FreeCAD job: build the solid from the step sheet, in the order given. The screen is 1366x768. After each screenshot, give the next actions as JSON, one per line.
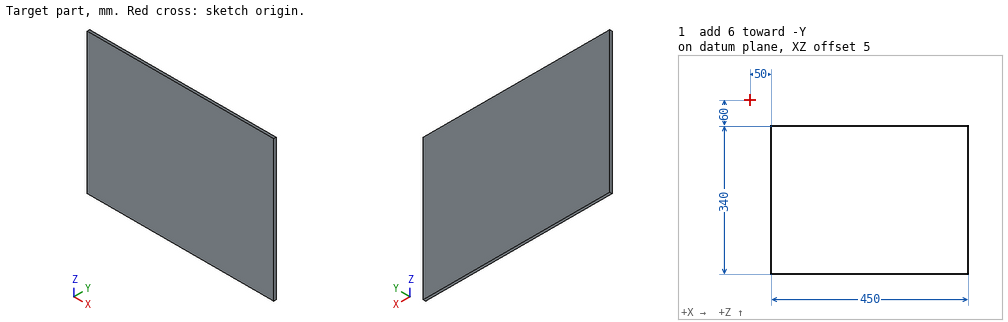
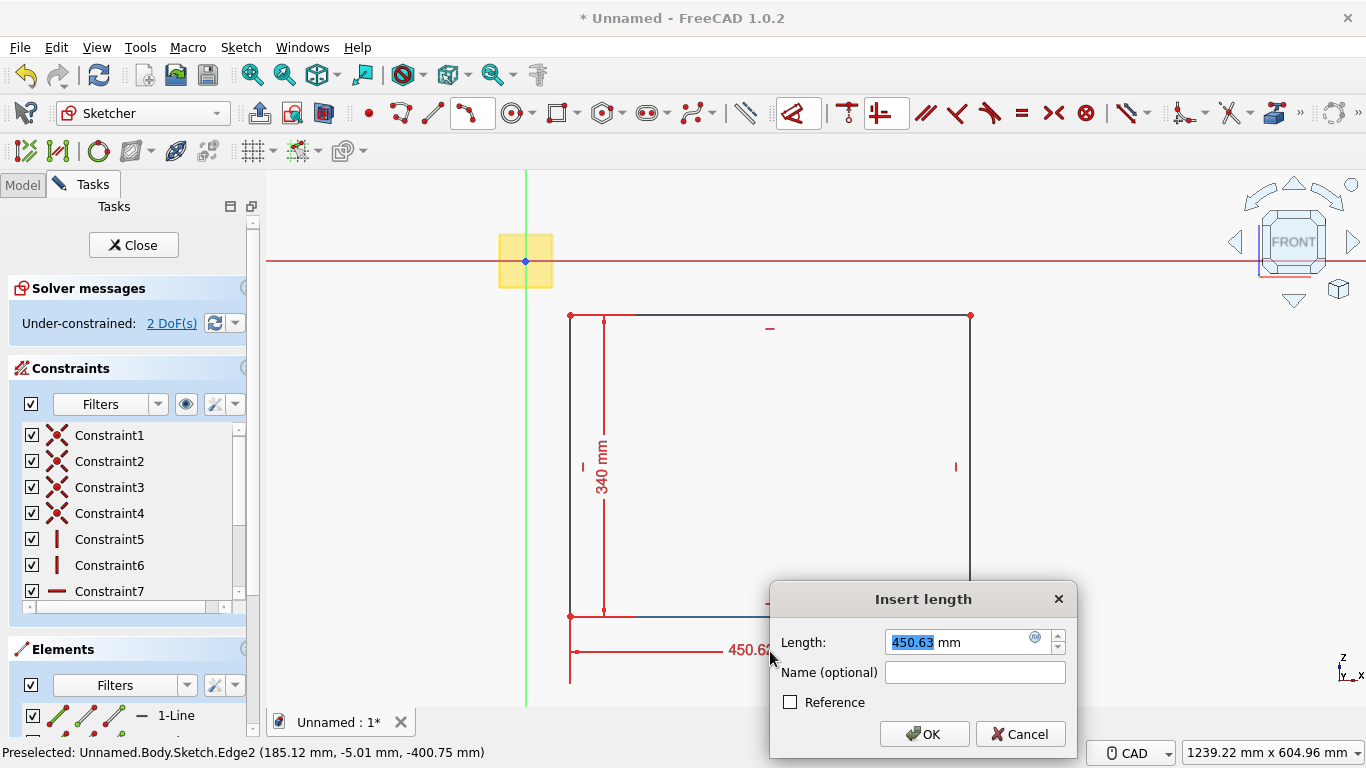
{"action": "type", "text": "450"}
{"action": "key", "text": "Return"}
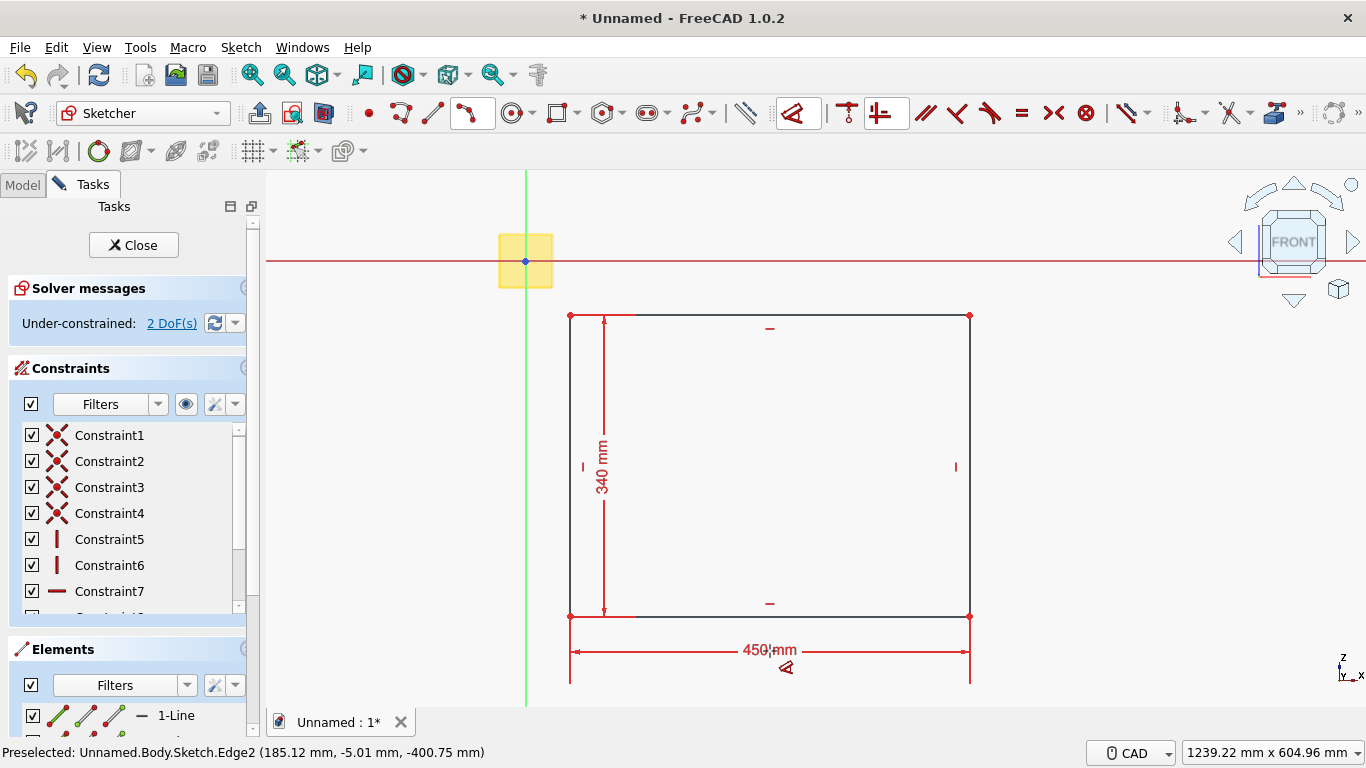
{"action": "left_click", "coordinate": [570, 315]}
{"action": "left_click", "coordinate": [548, 227]}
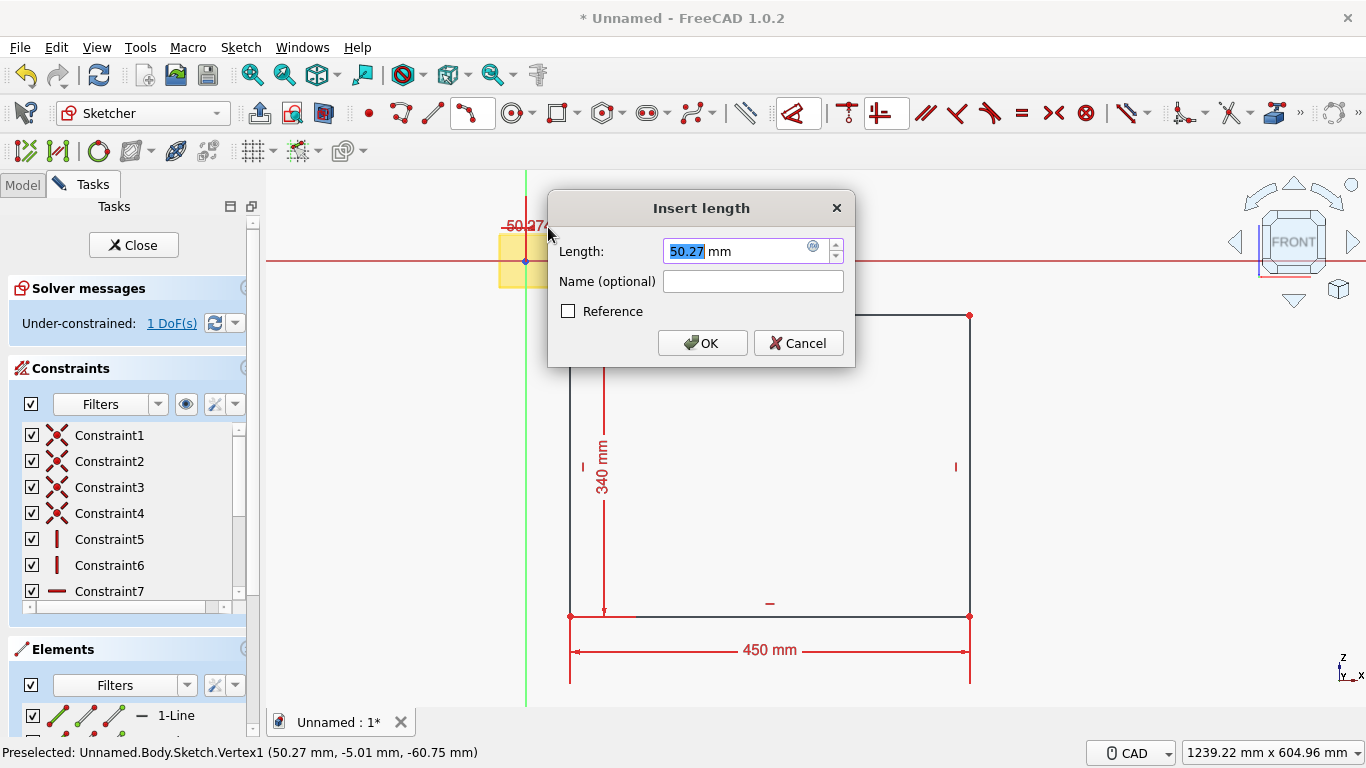
{"action": "type", "text": "50"}
{"action": "key", "text": "Return"}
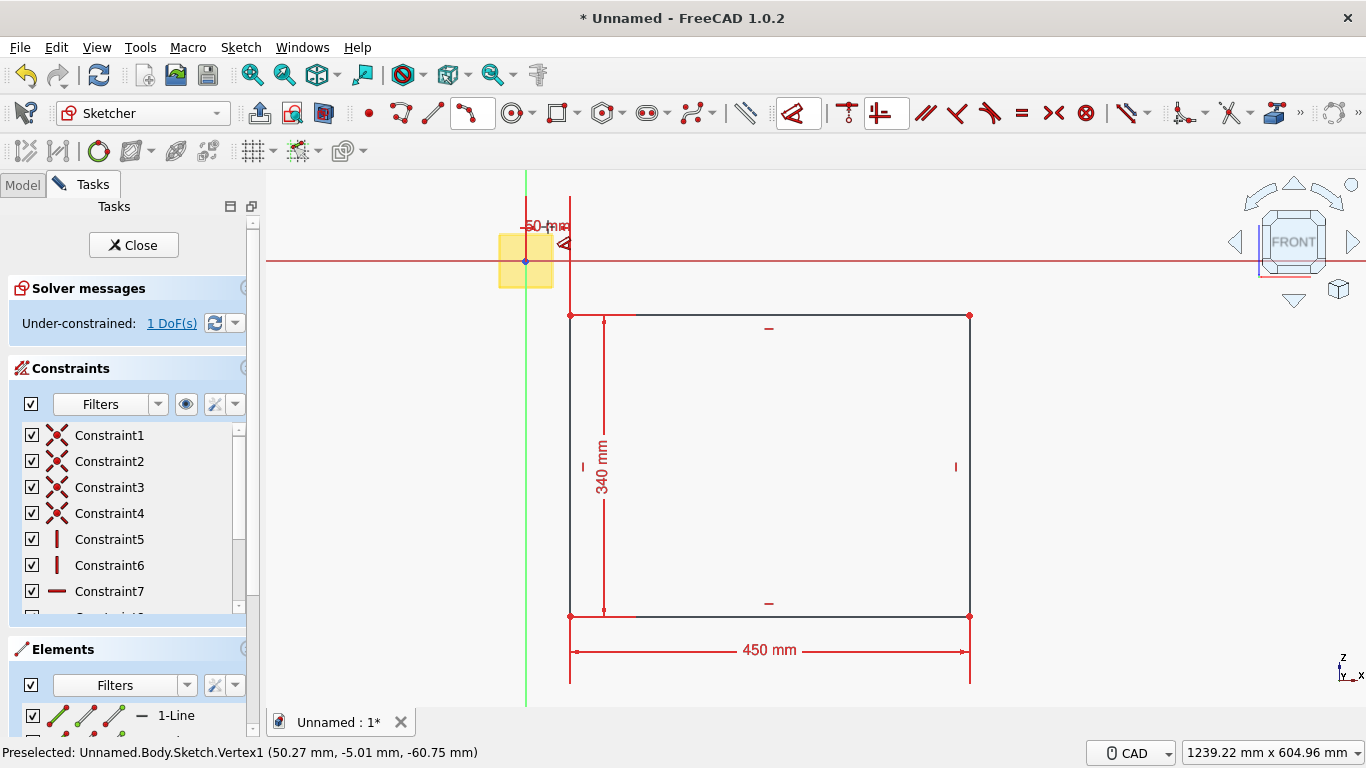
{"action": "left_click", "coordinate": [570, 315]}
{"action": "left_click", "coordinate": [492, 288]}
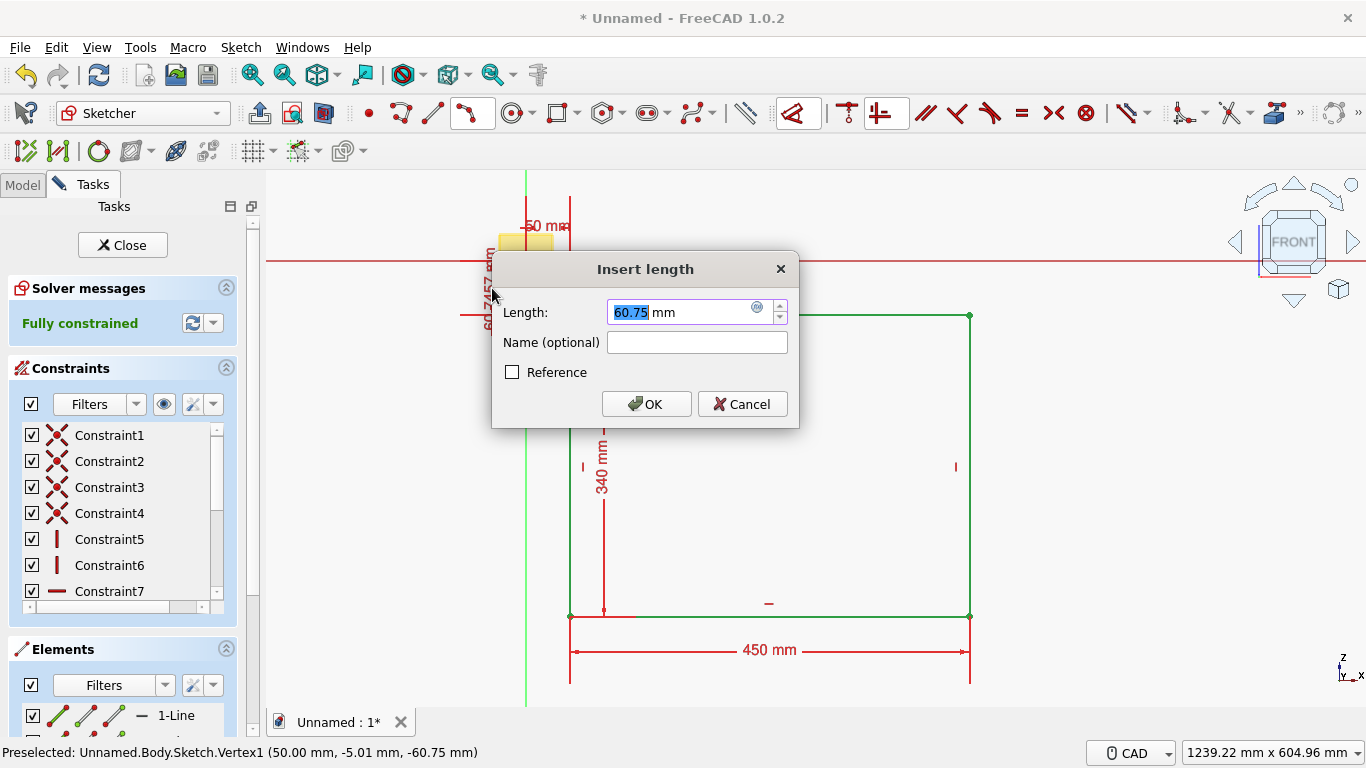
{"action": "type", "text": "60"}
{"action": "key", "text": "Return"}
{"action": "key", "text": "Escape"}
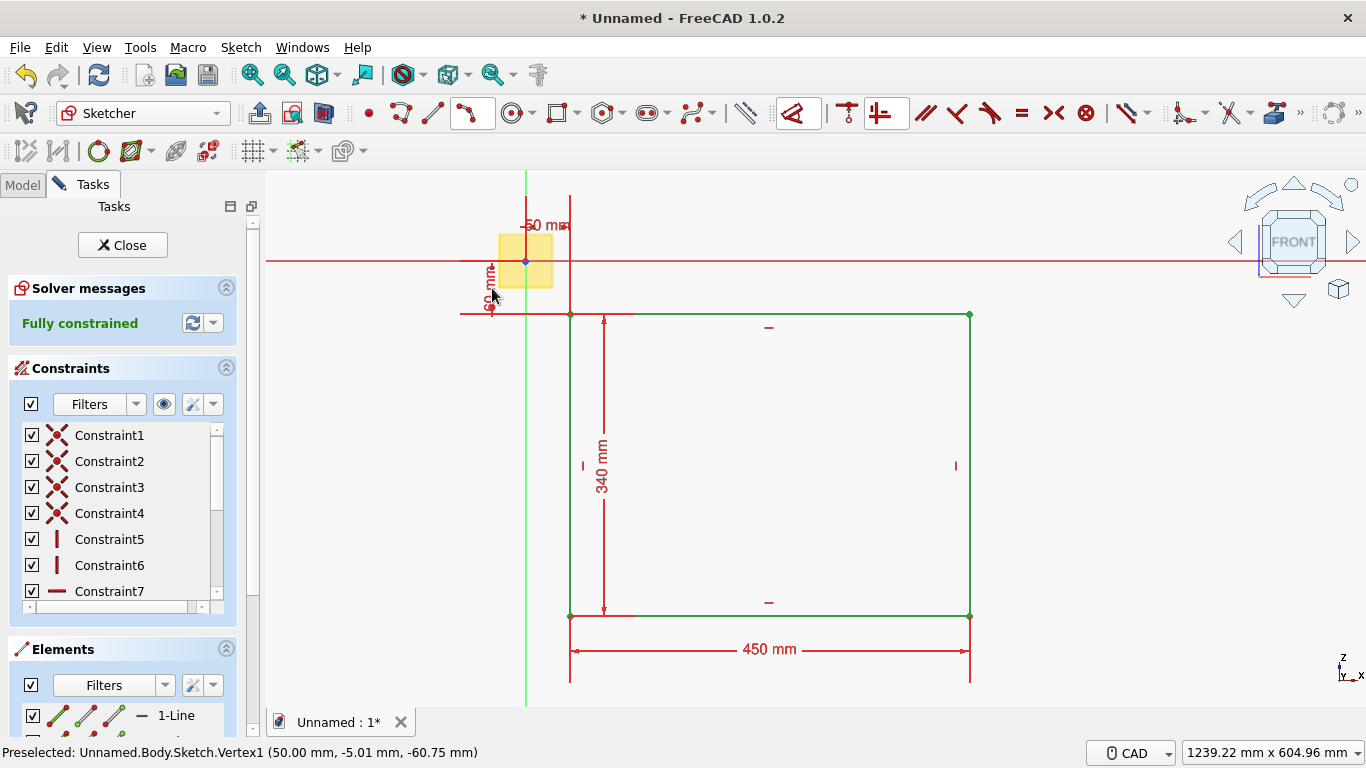
{"action": "left_click", "coordinate": [123, 245]}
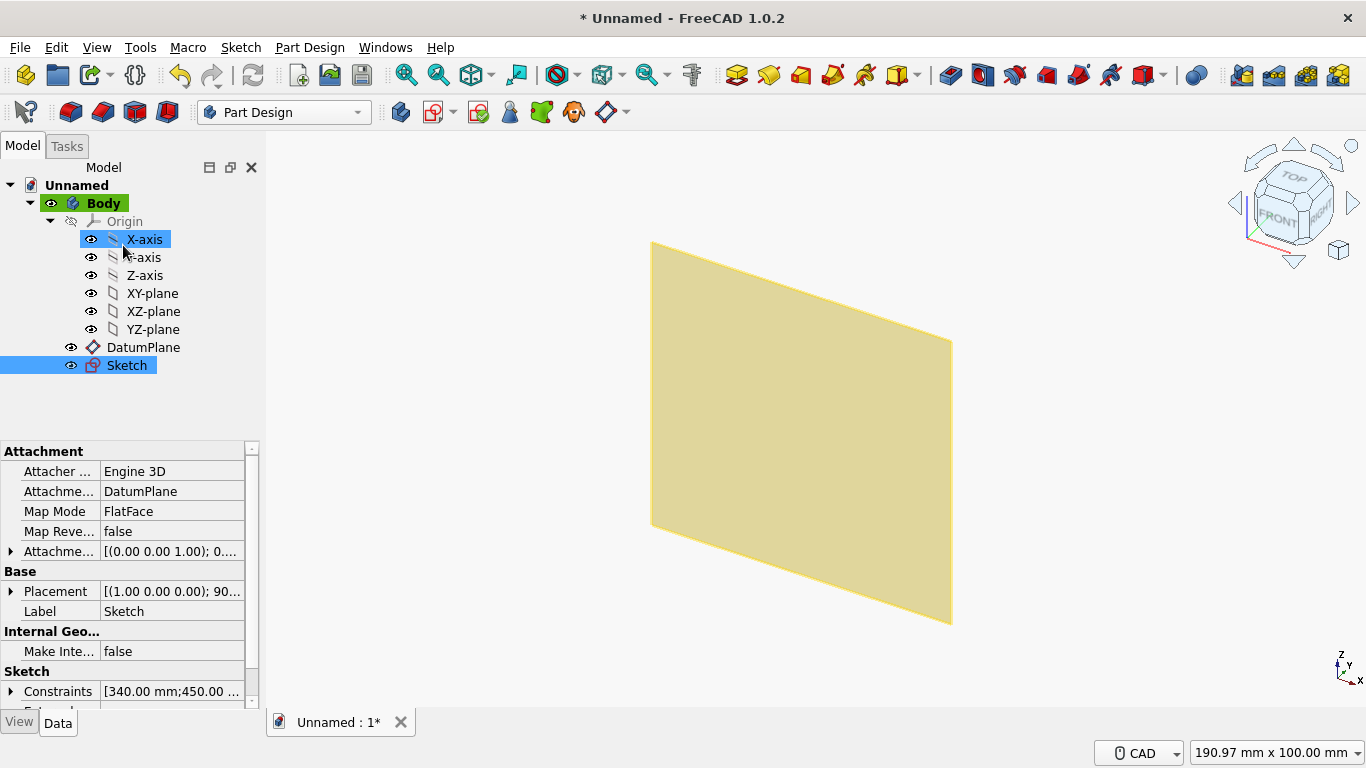
{"action": "left_click", "coordinate": [738, 76]}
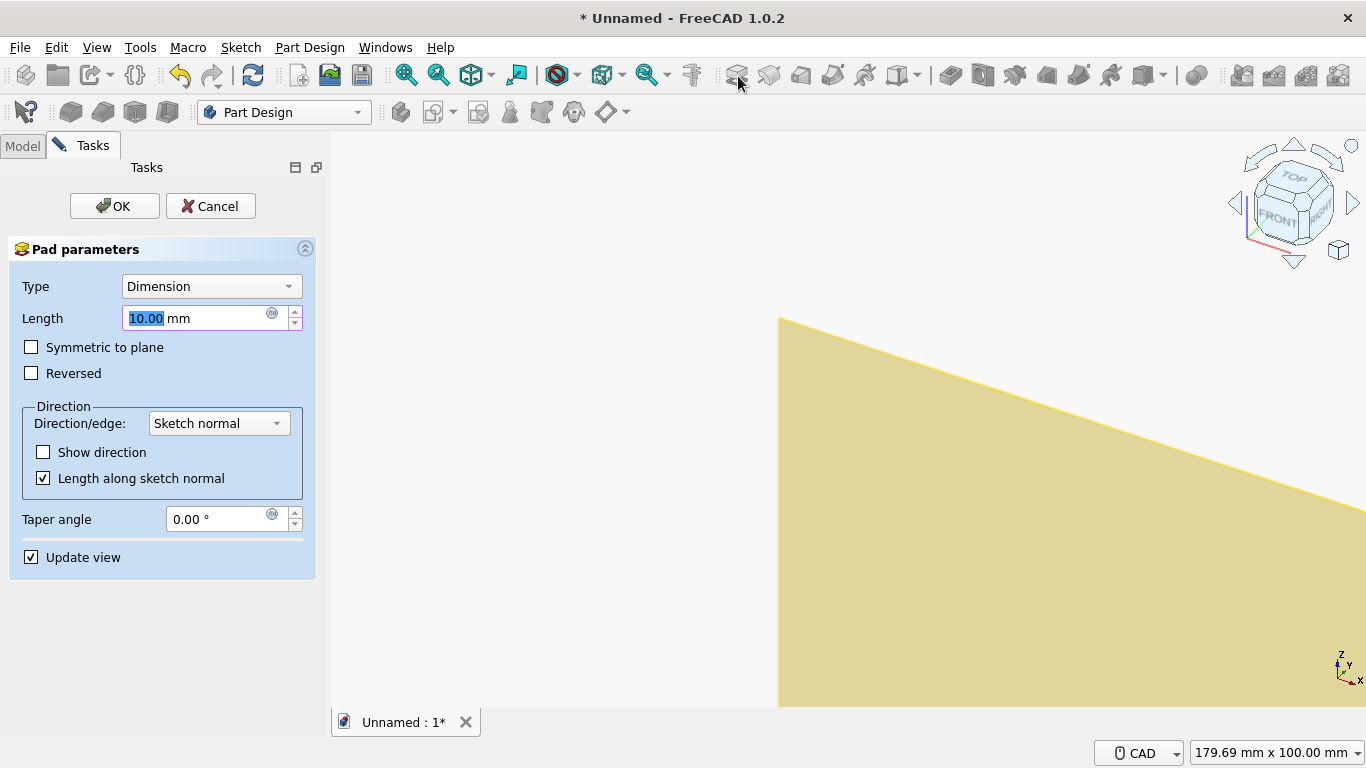
{"action": "type", "text": "6"}
{"action": "key", "text": "Tab"}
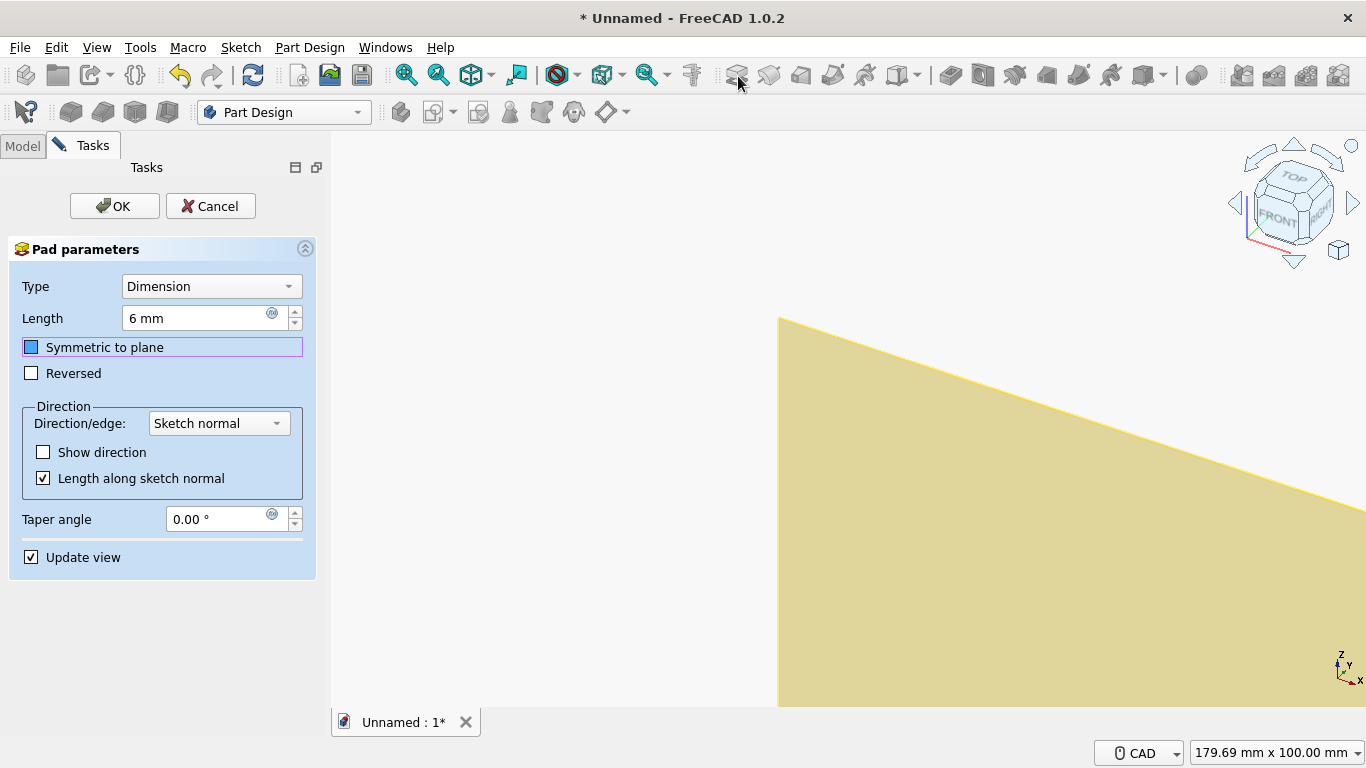
{"action": "left_click", "coordinate": [115, 206]}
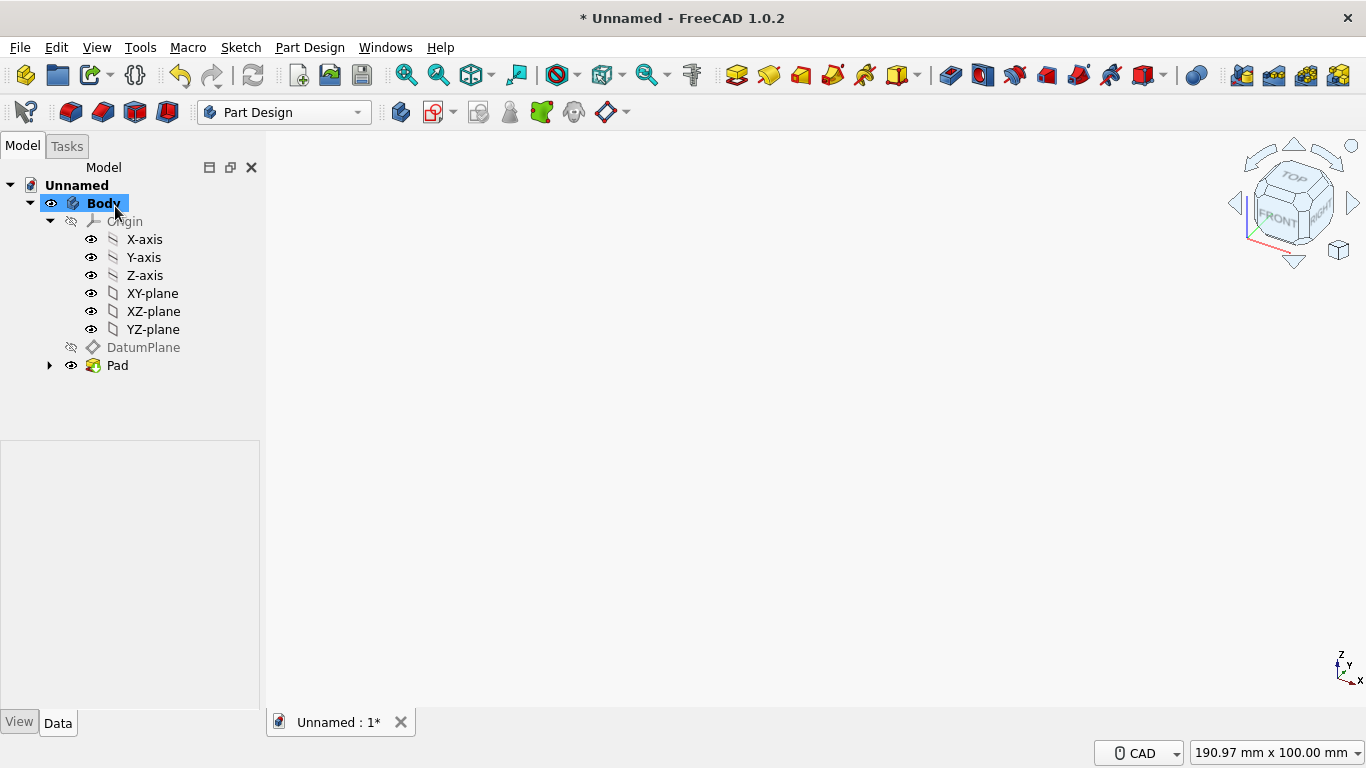
{"action": "key", "text": "0"}